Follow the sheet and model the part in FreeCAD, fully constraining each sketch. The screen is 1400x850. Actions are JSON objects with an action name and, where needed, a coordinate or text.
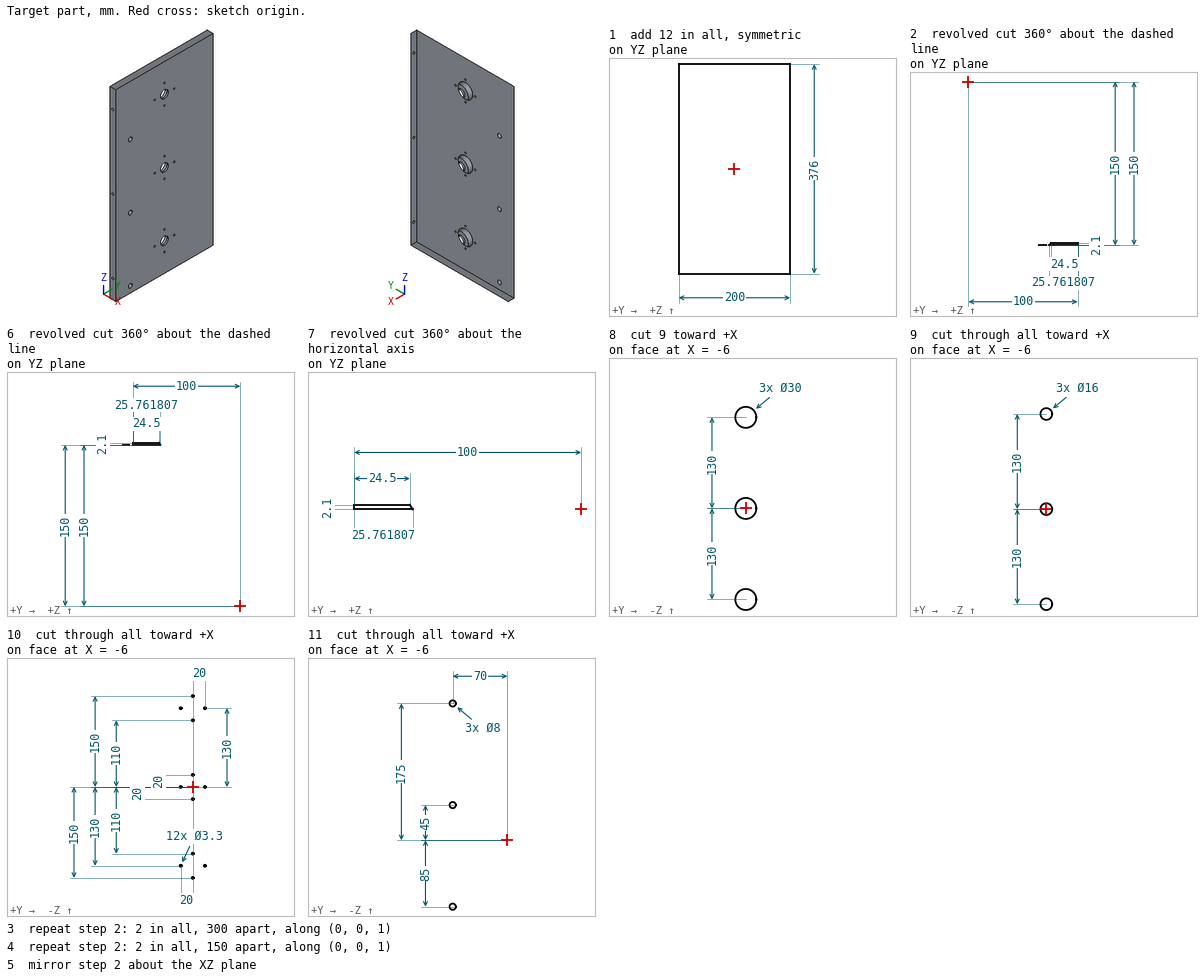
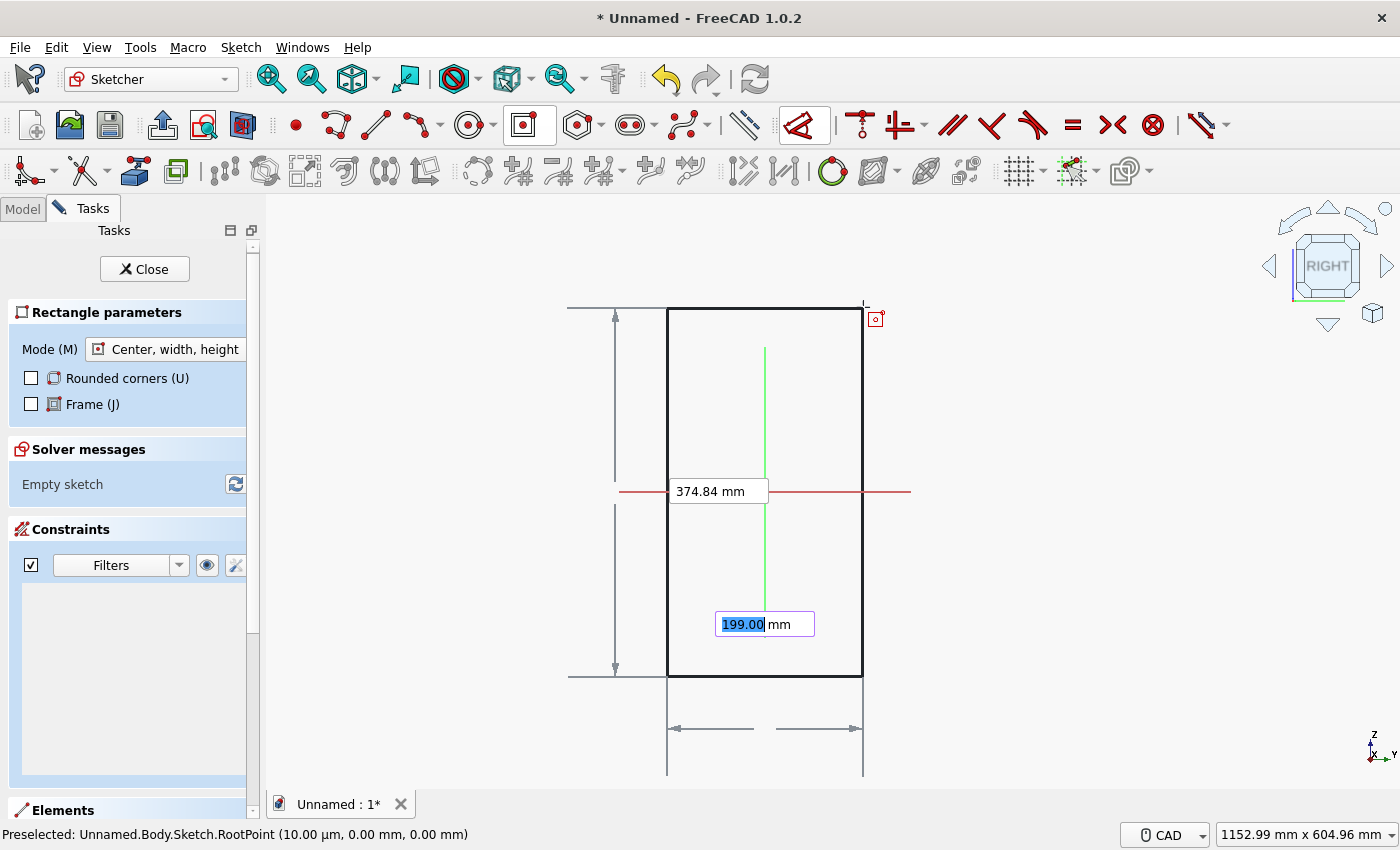
{"action": "type", "text": "200"}
{"action": "key", "text": "Tab"}
{"action": "type", "text": "376"}
{"action": "key", "text": "Return"}
{"action": "key", "text": "Escape"}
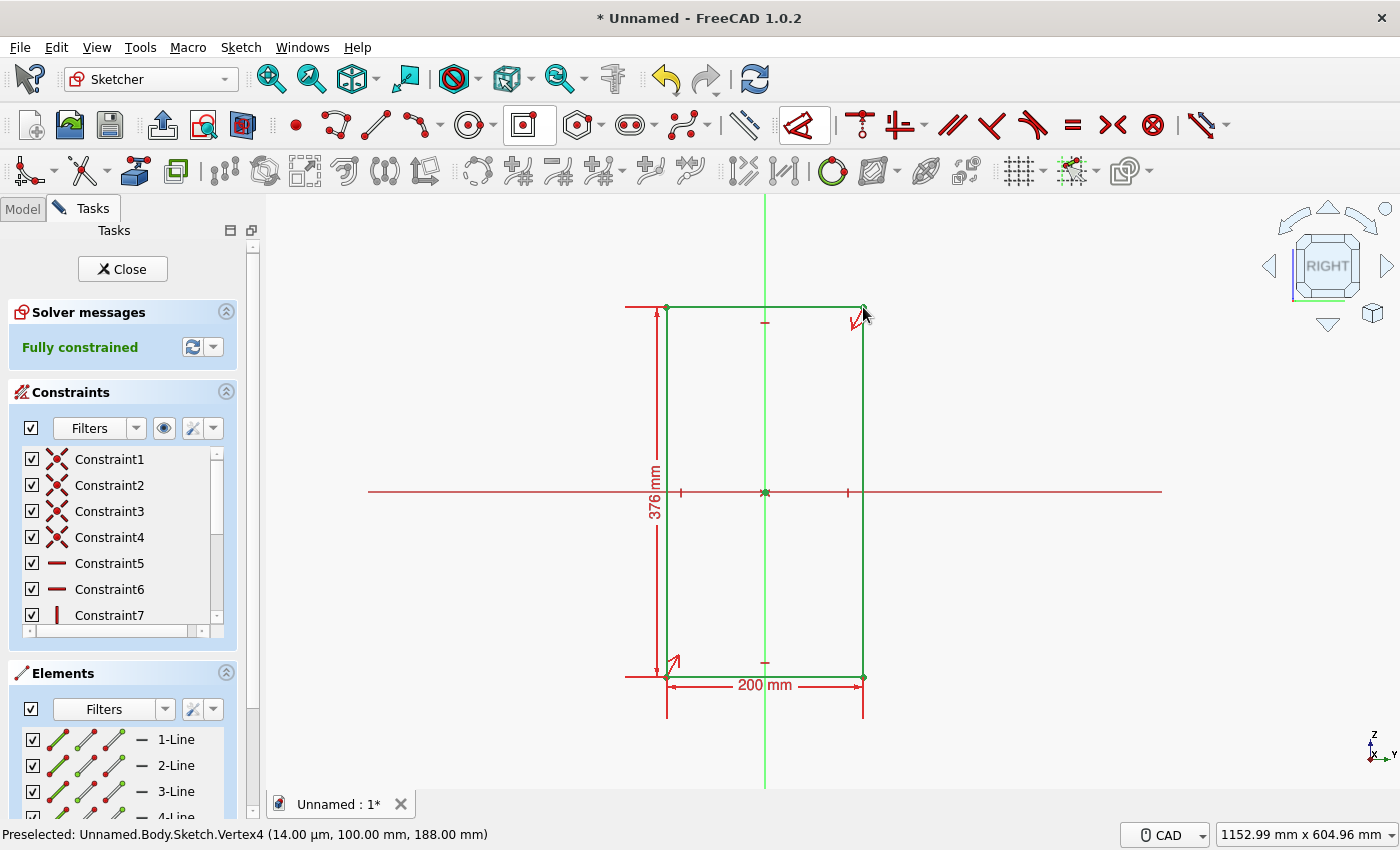
{"action": "left_click", "coordinate": [123, 269]}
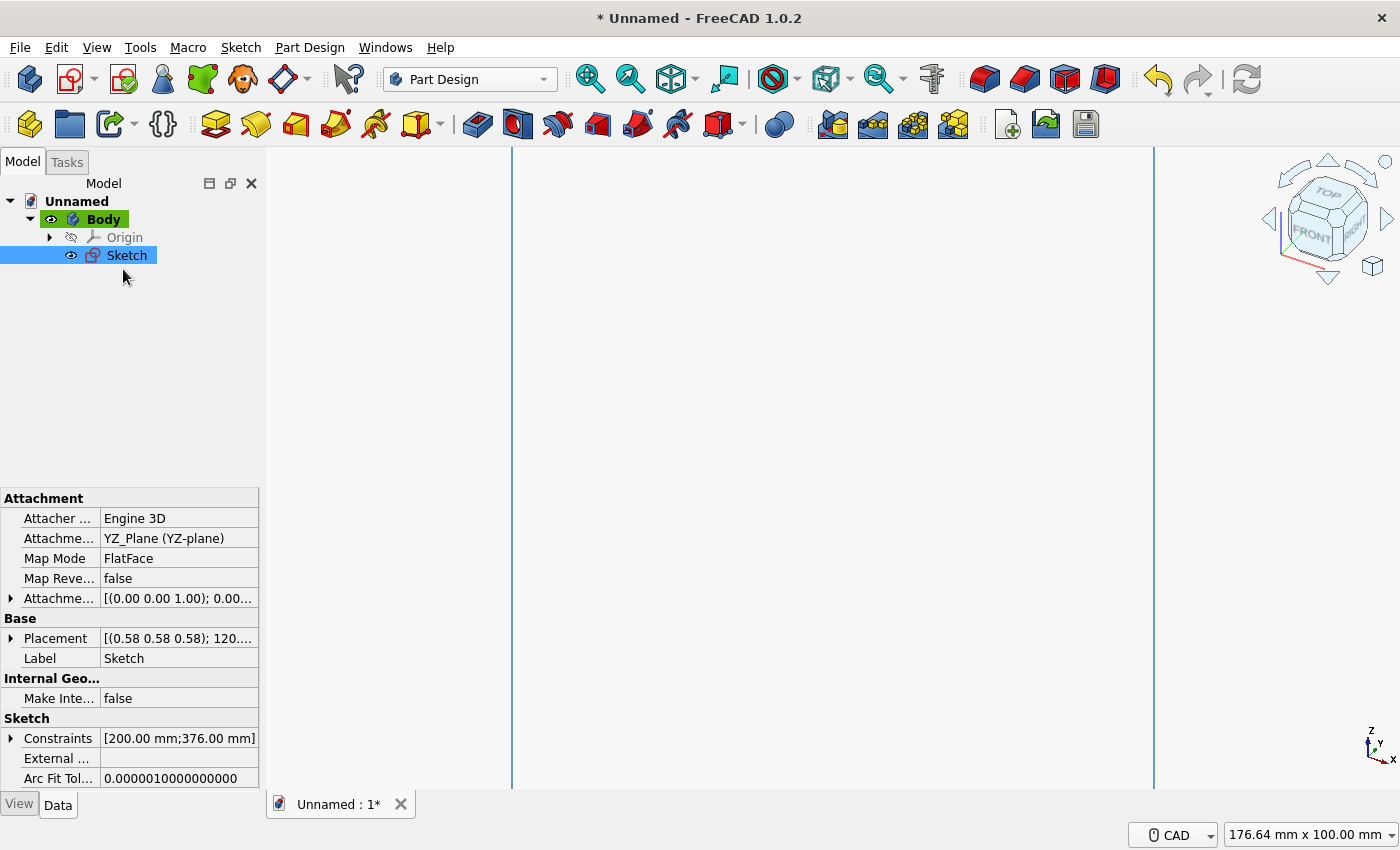
{"action": "left_click", "coordinate": [216, 124]}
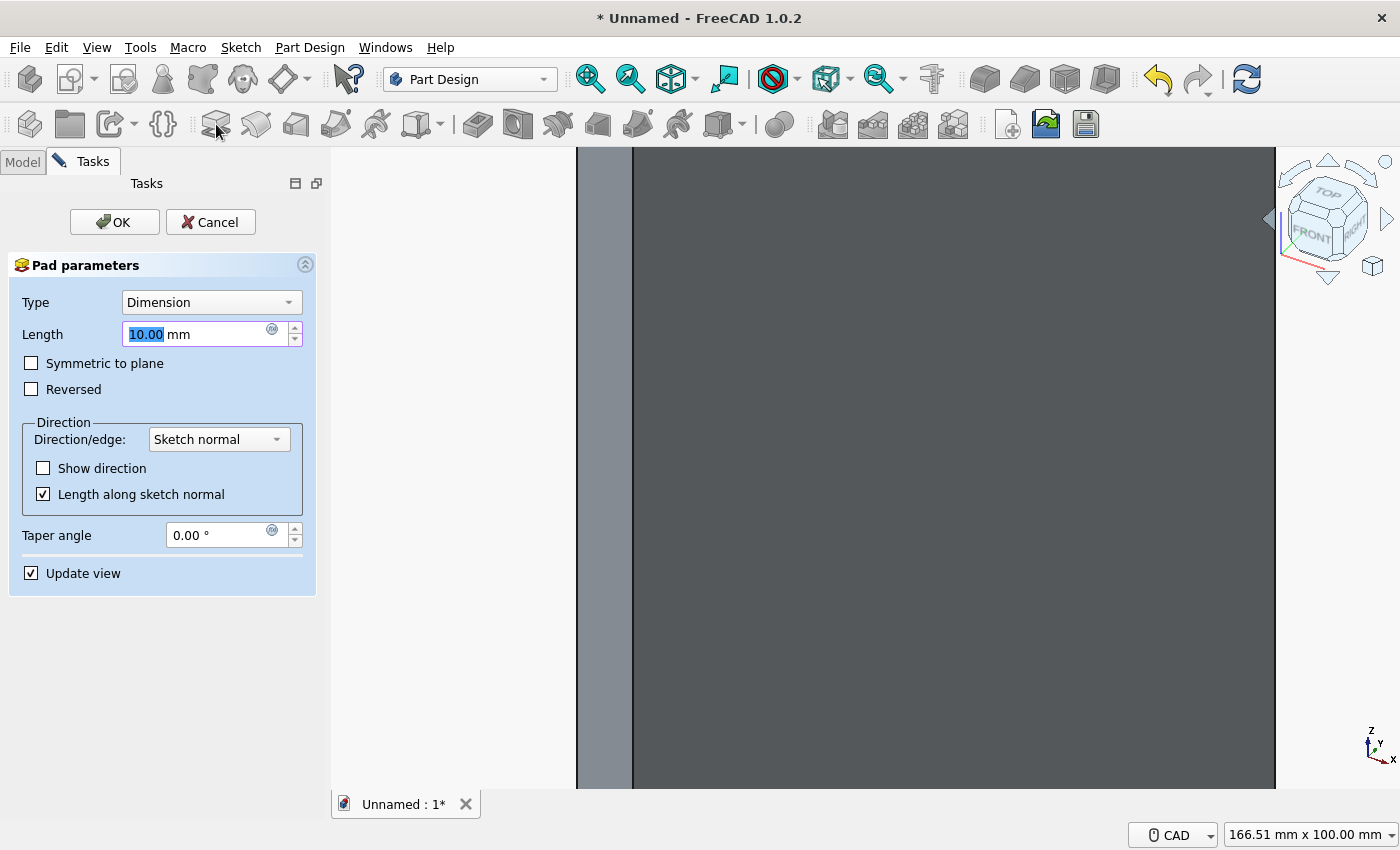
{"action": "type", "text": "12"}
{"action": "key", "text": "Tab"}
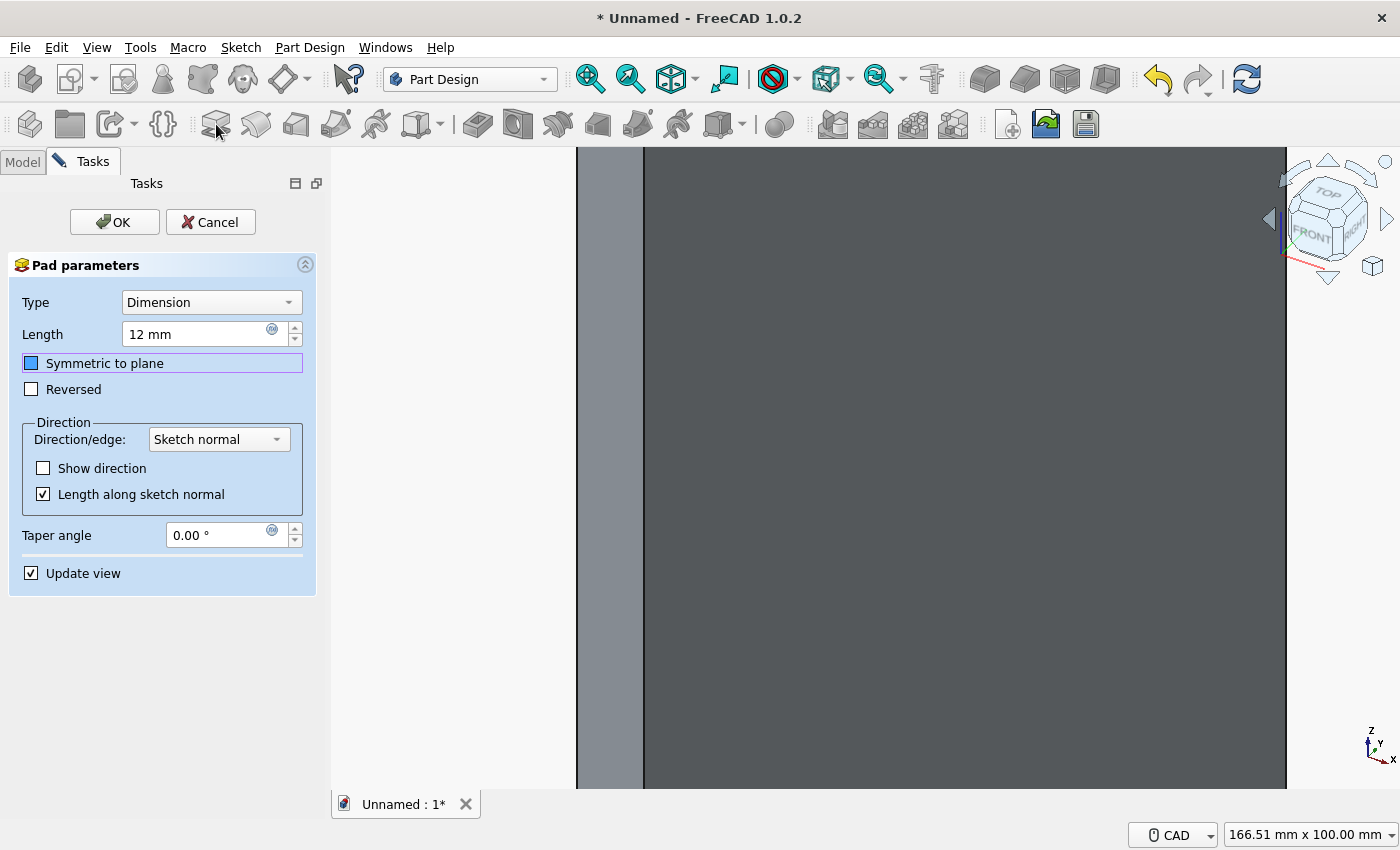
{"action": "left_click", "coordinate": [30, 363]}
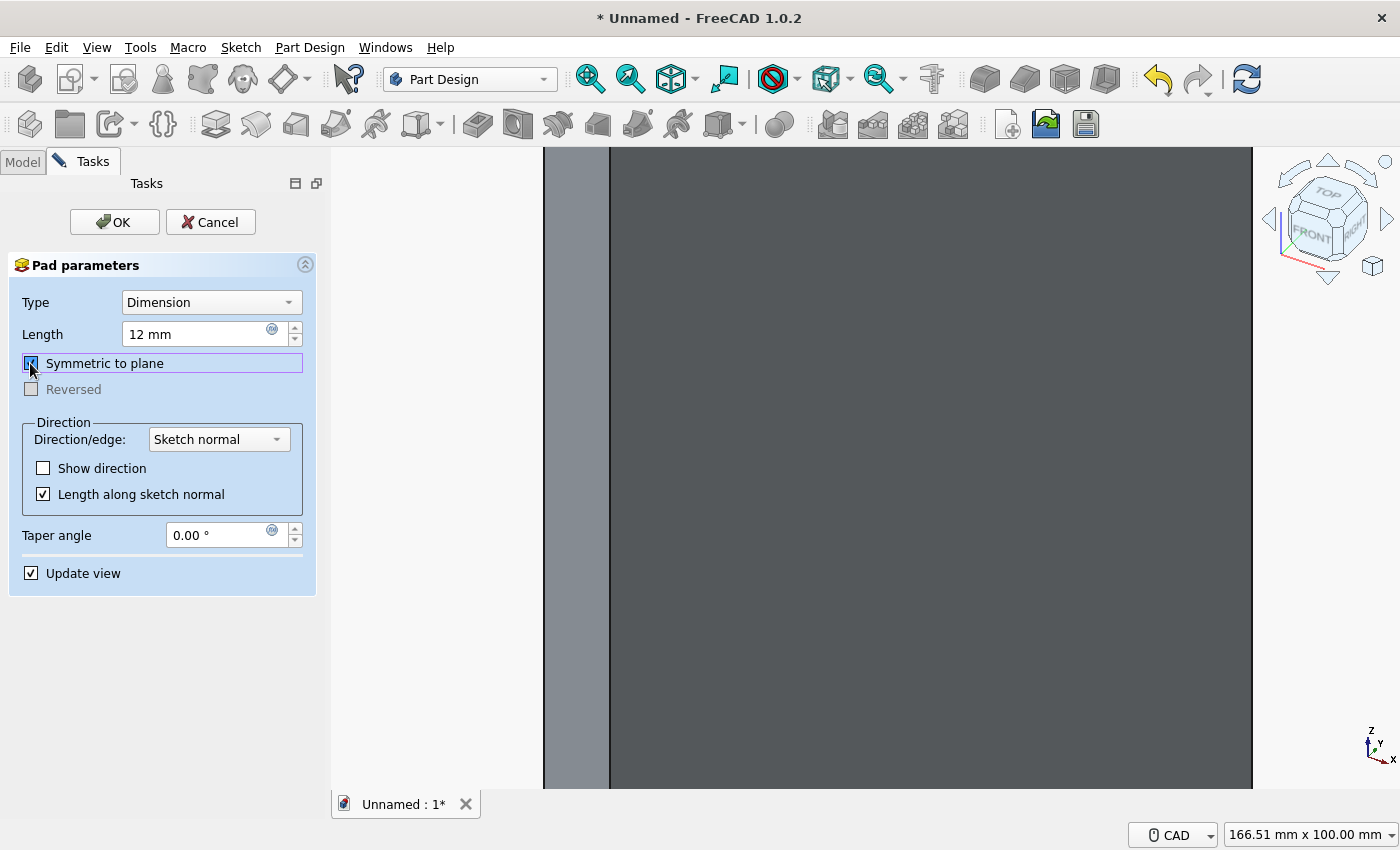
{"action": "left_click", "coordinate": [115, 222]}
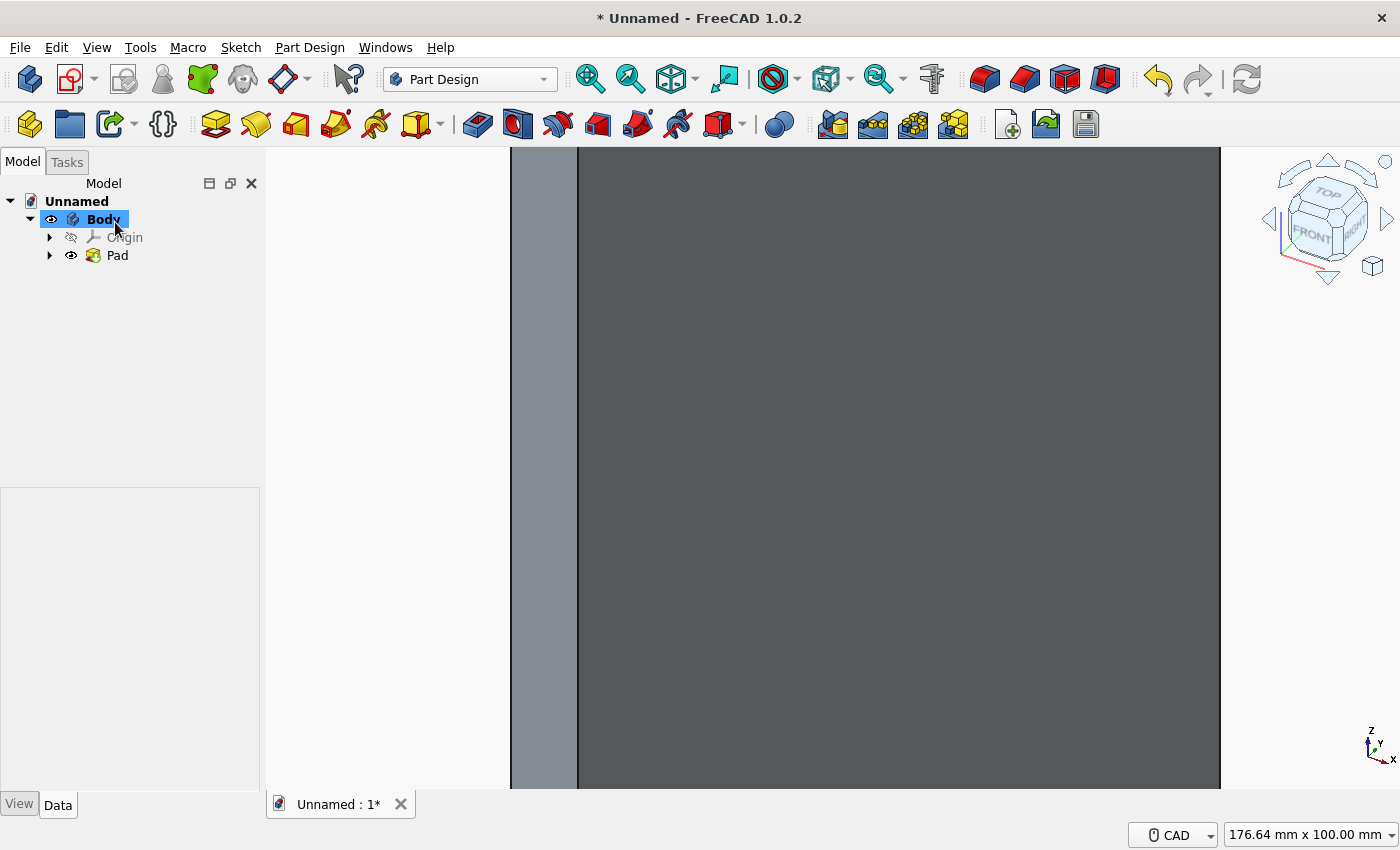
{"action": "left_click", "coordinate": [592, 80]}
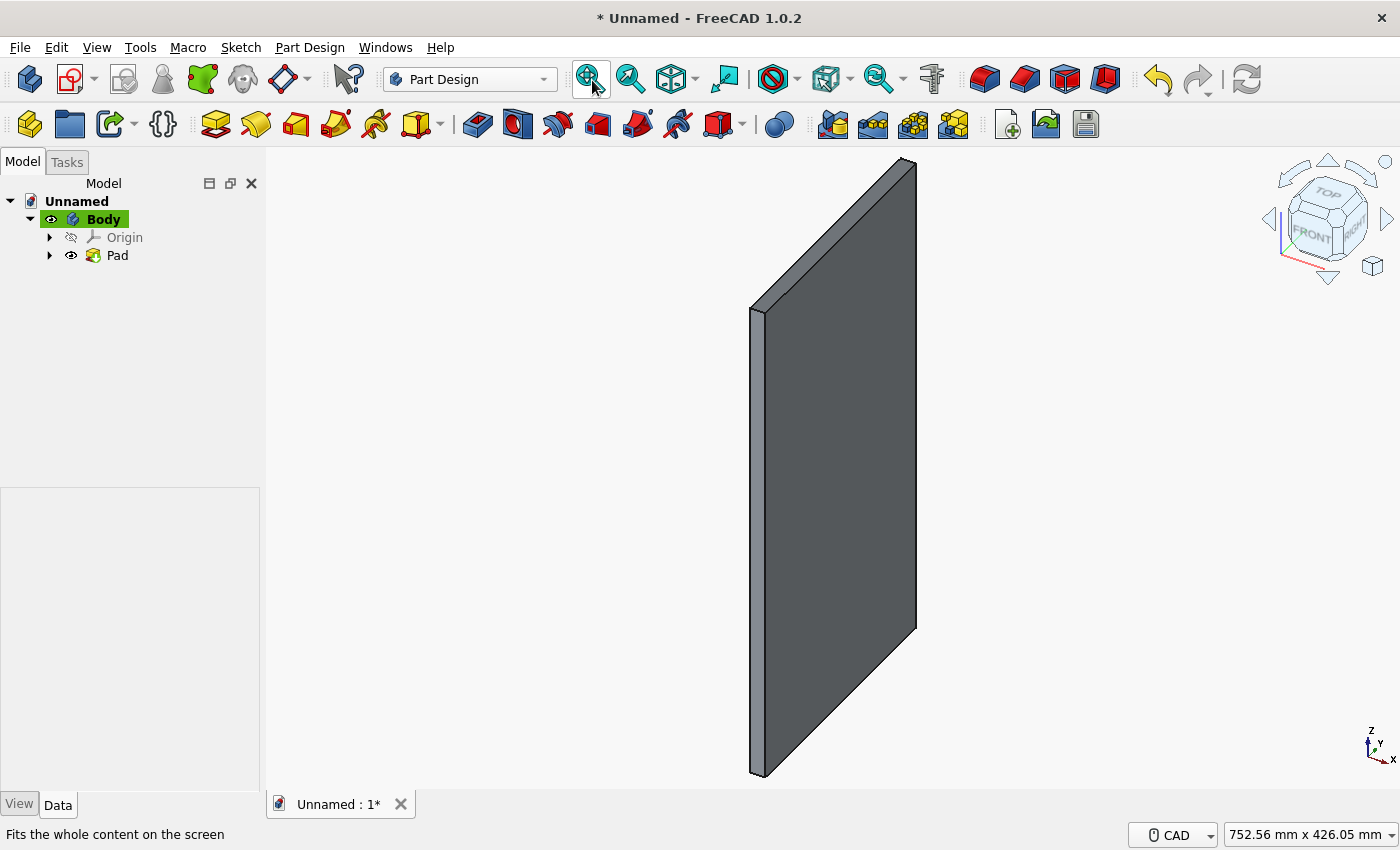
{"action": "left_click", "coordinate": [70, 80]}